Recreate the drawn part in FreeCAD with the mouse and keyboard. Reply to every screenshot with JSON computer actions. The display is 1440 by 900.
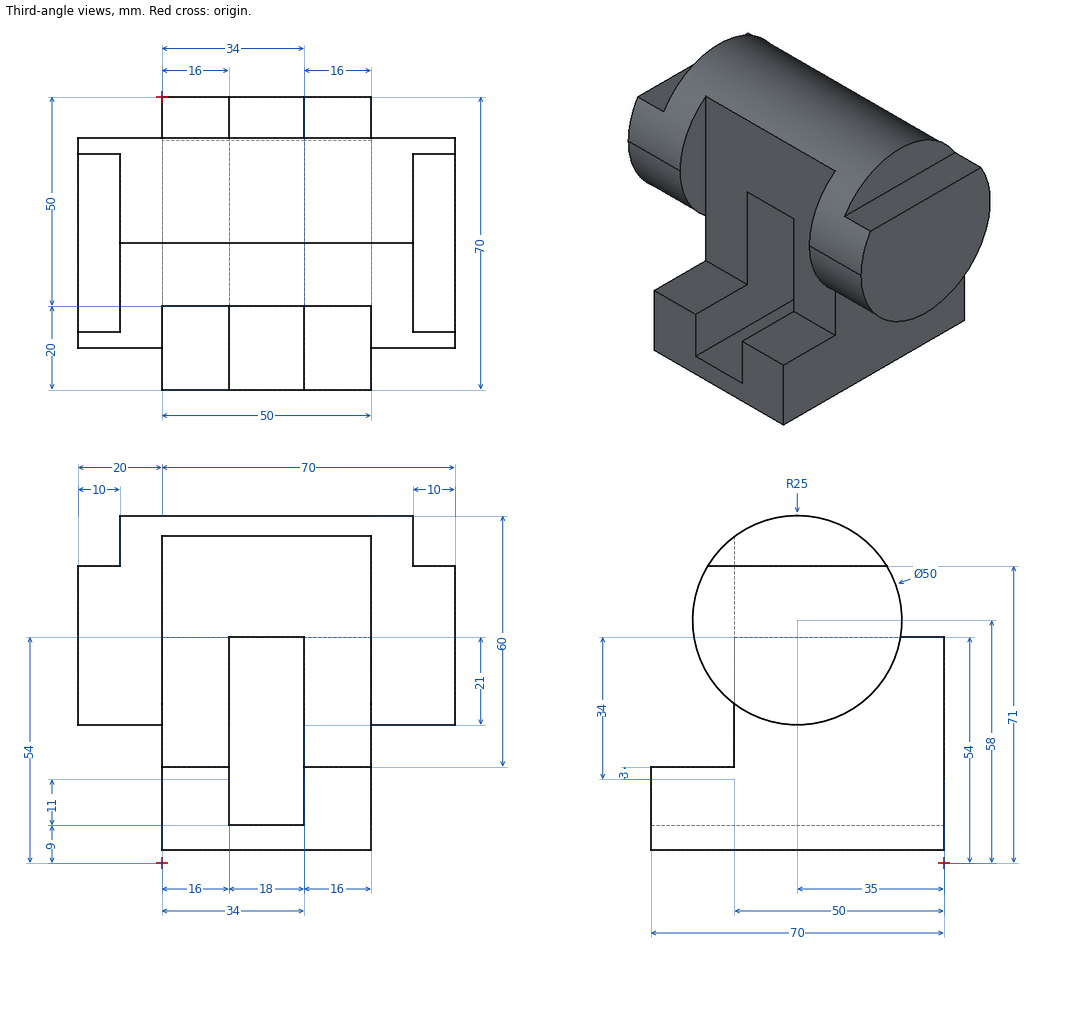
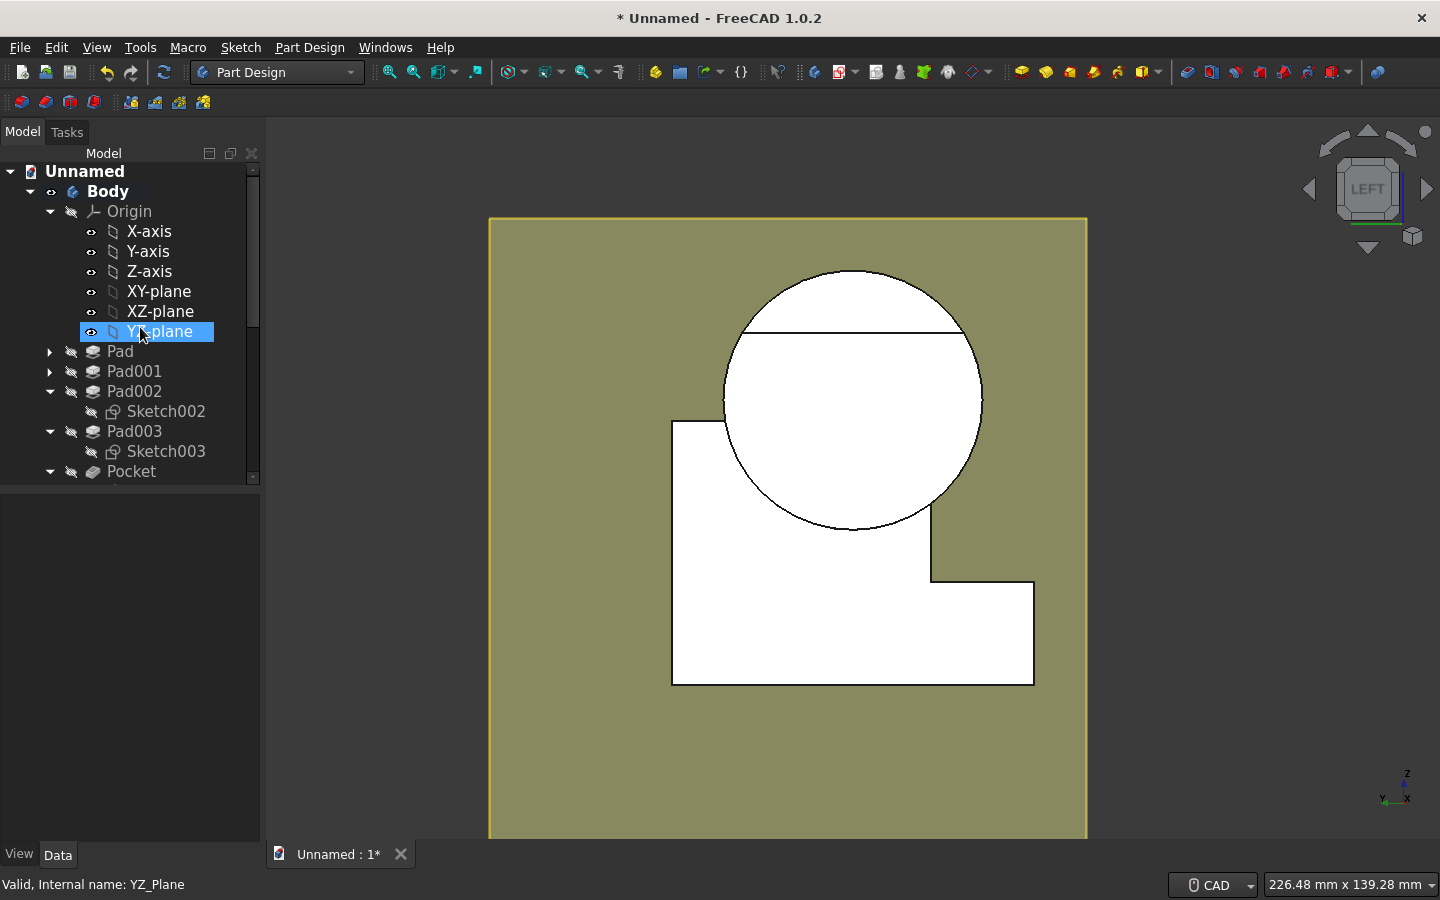
{"action": "scroll", "coordinate": [100, 327], "scroll_direction": "down", "scroll_amount": 6}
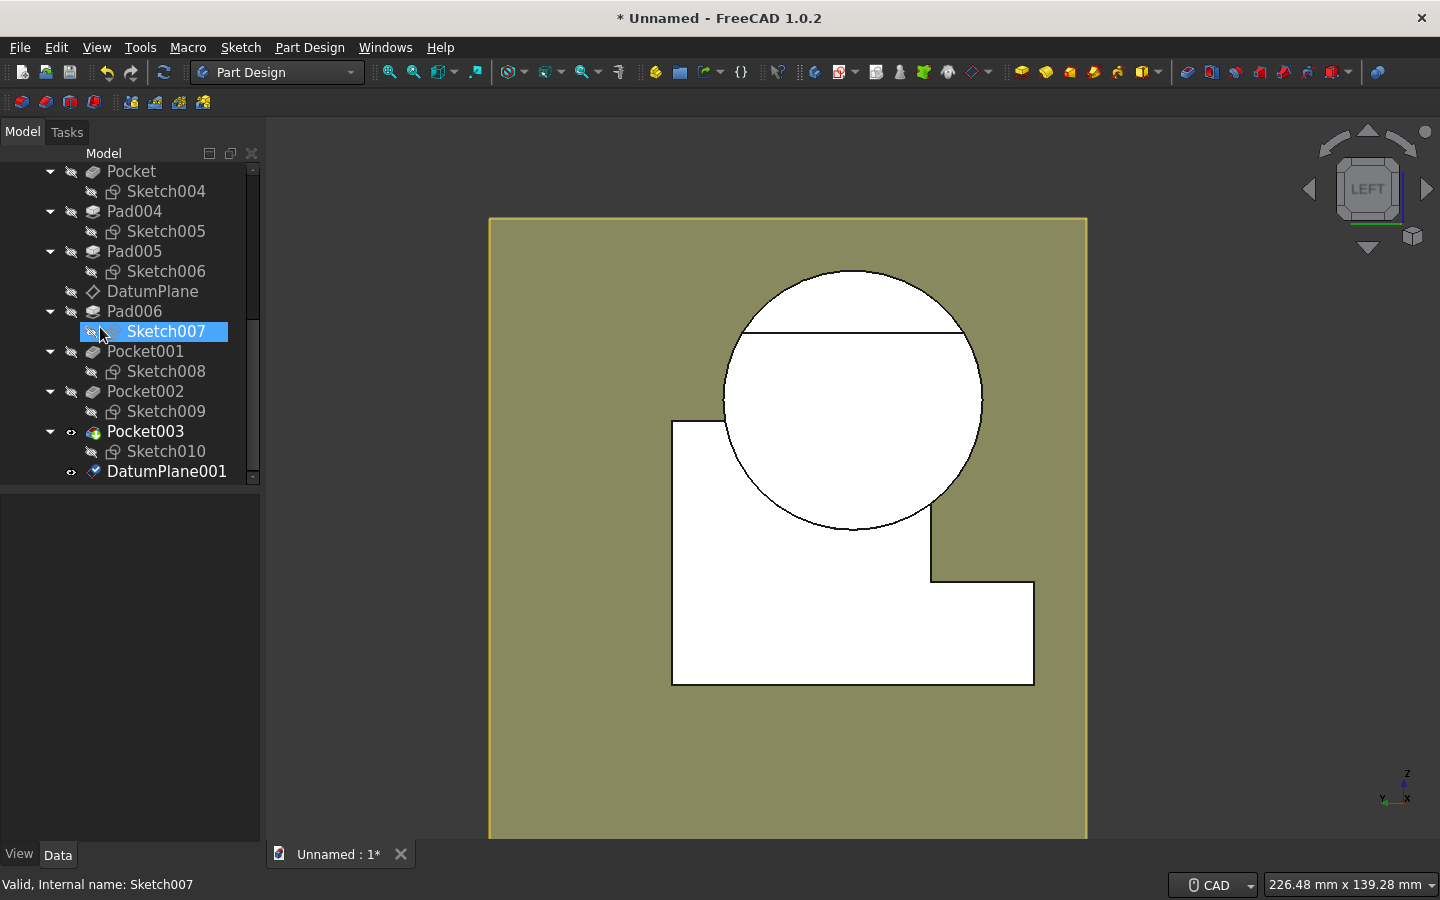
{"action": "left_click", "coordinate": [116, 472]}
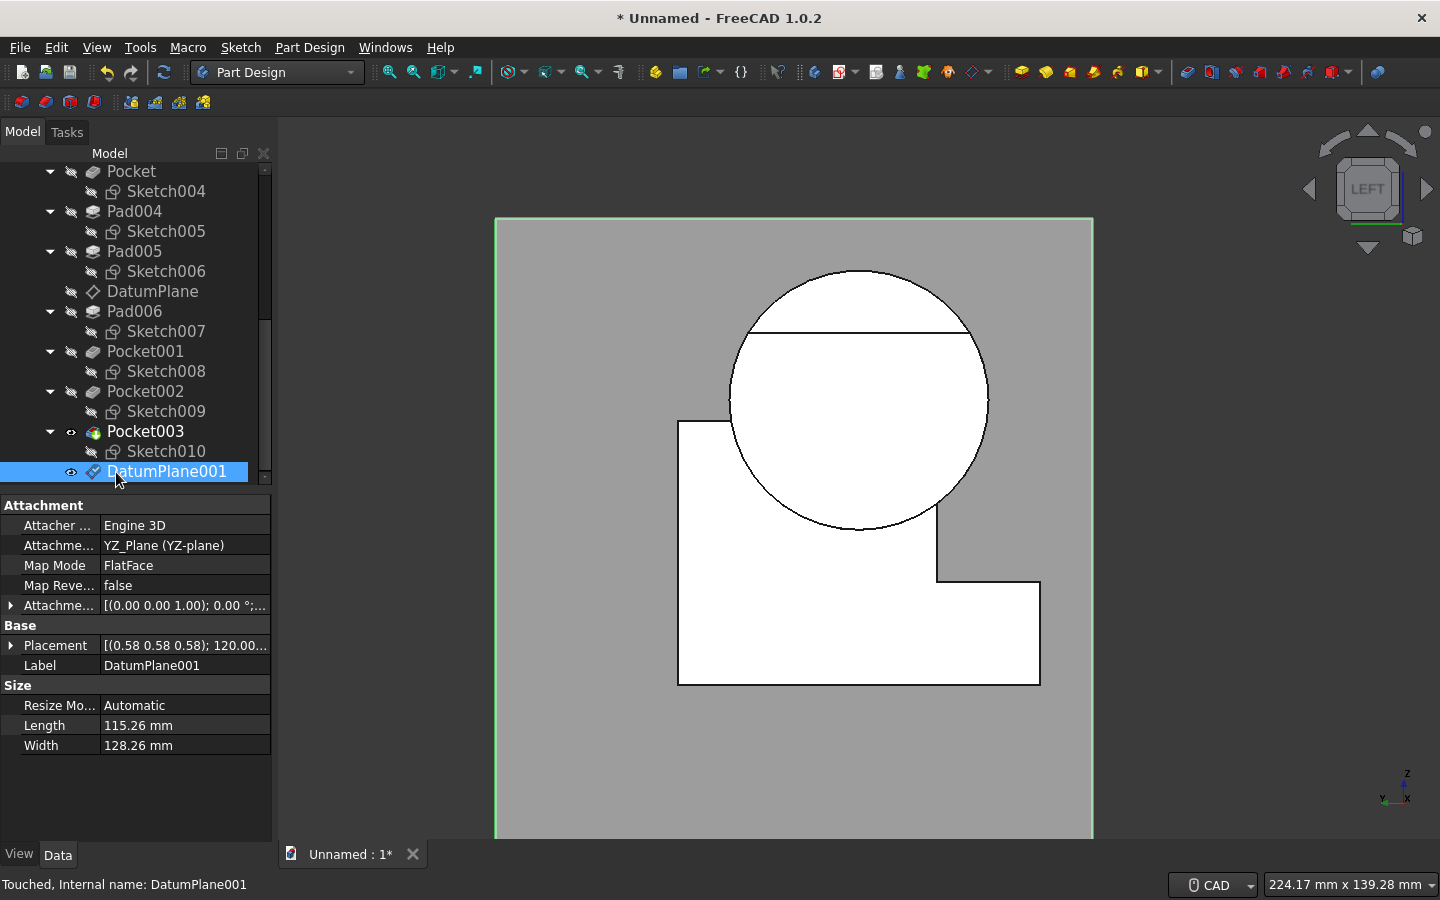
{"action": "left_click", "coordinate": [840, 72]}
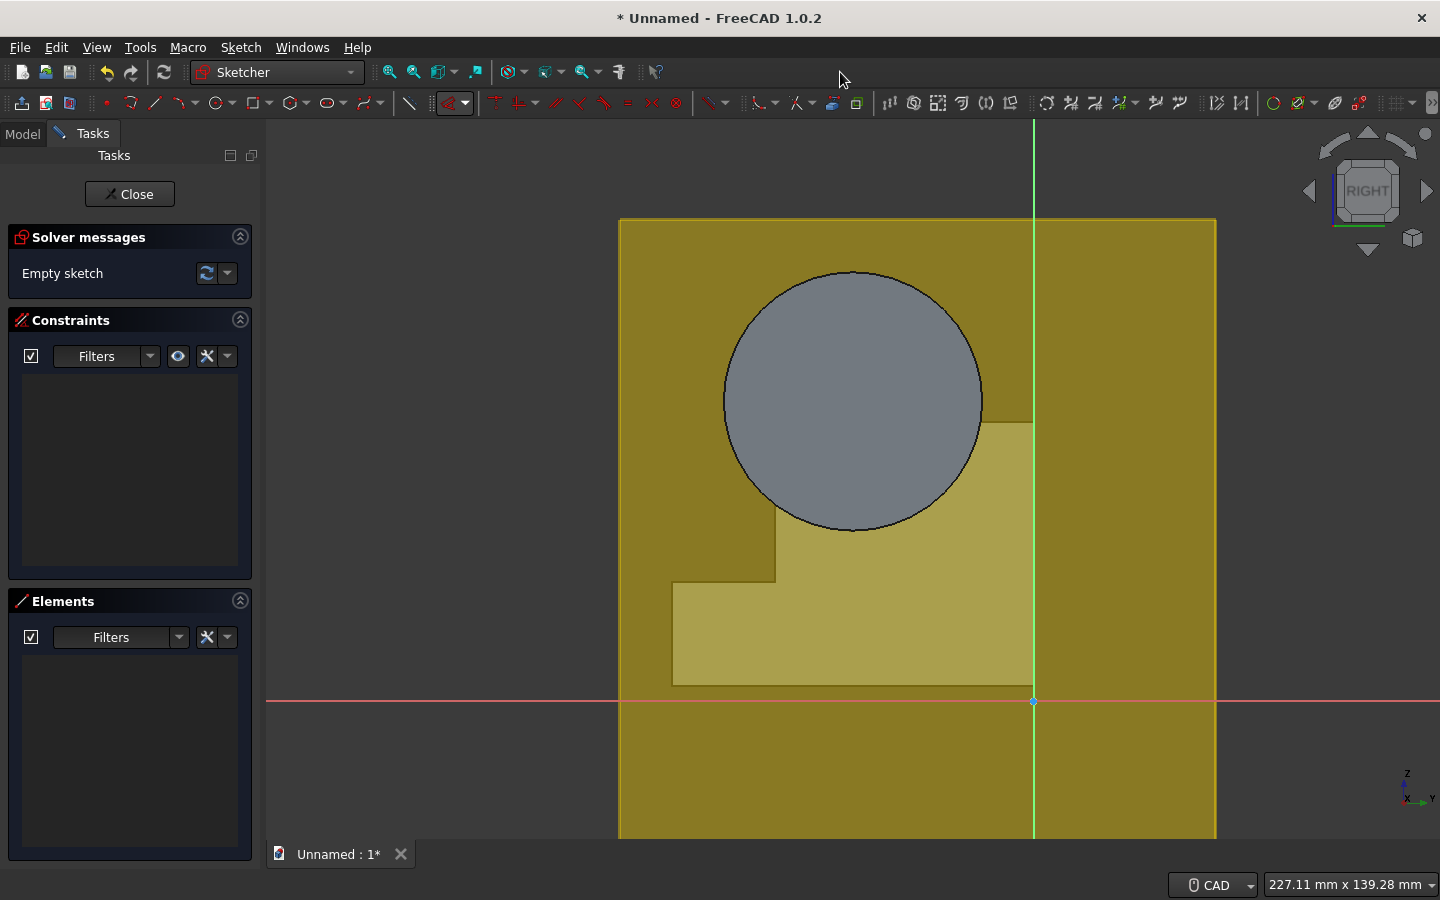
{"action": "key", "text": "q s"}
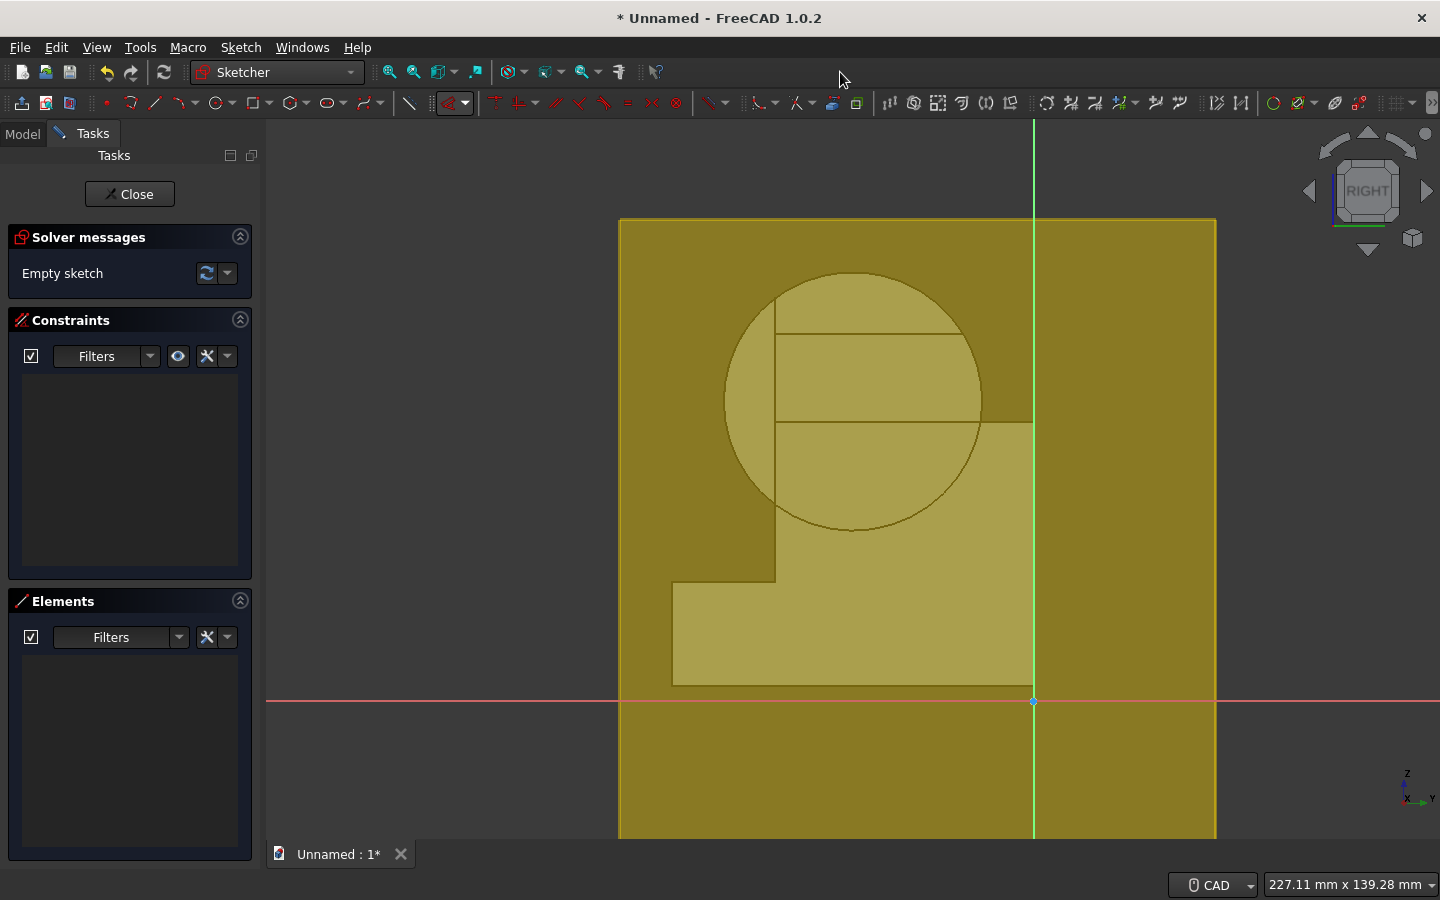
{"action": "key", "text": "g l"}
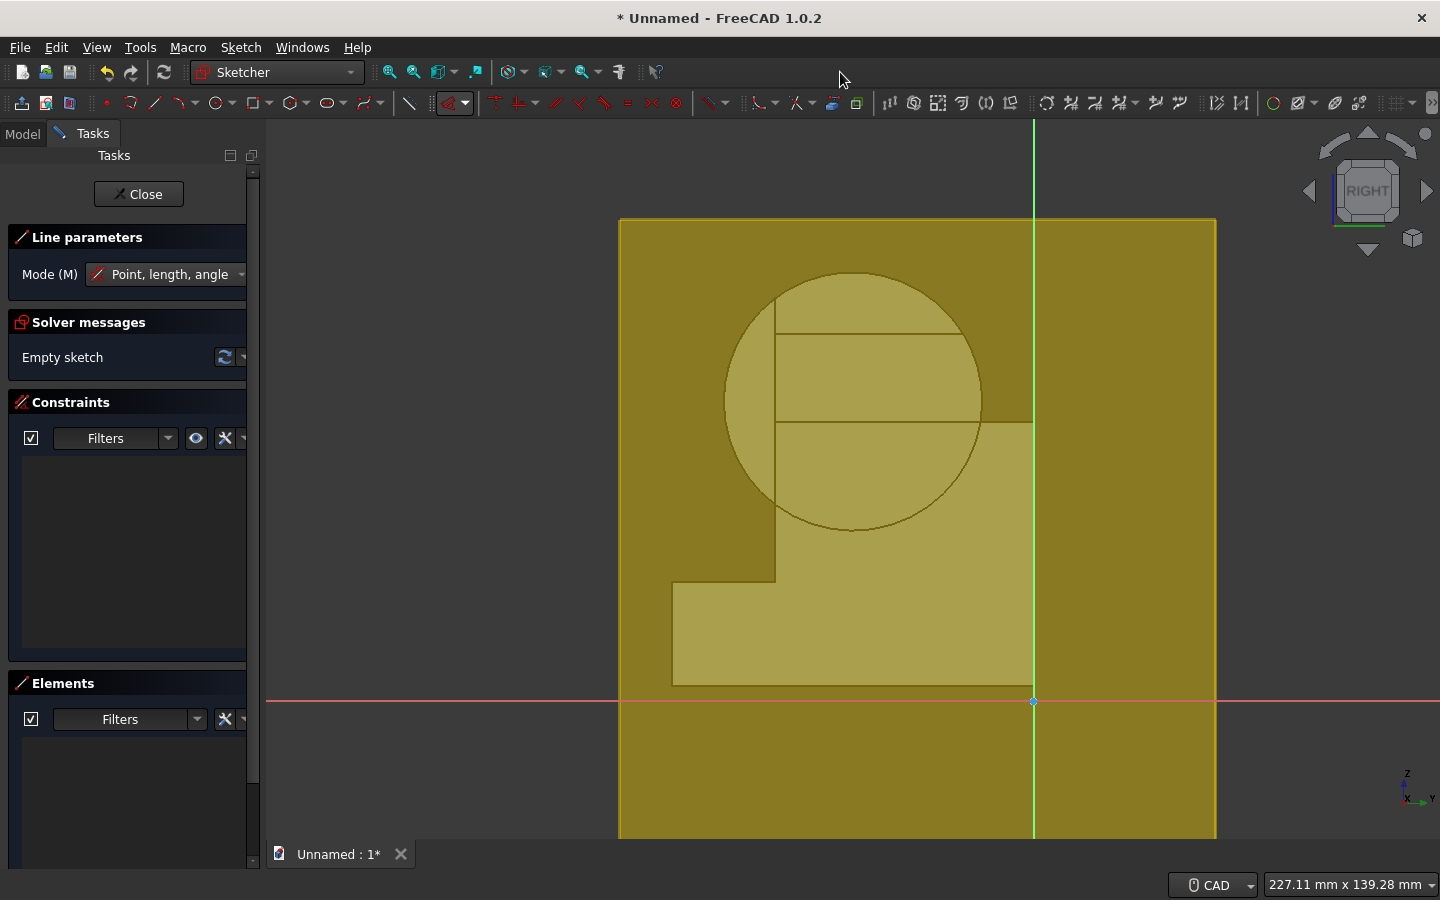
{"action": "left_click", "coordinate": [743, 334]}
{"action": "left_click", "coordinate": [963, 334]}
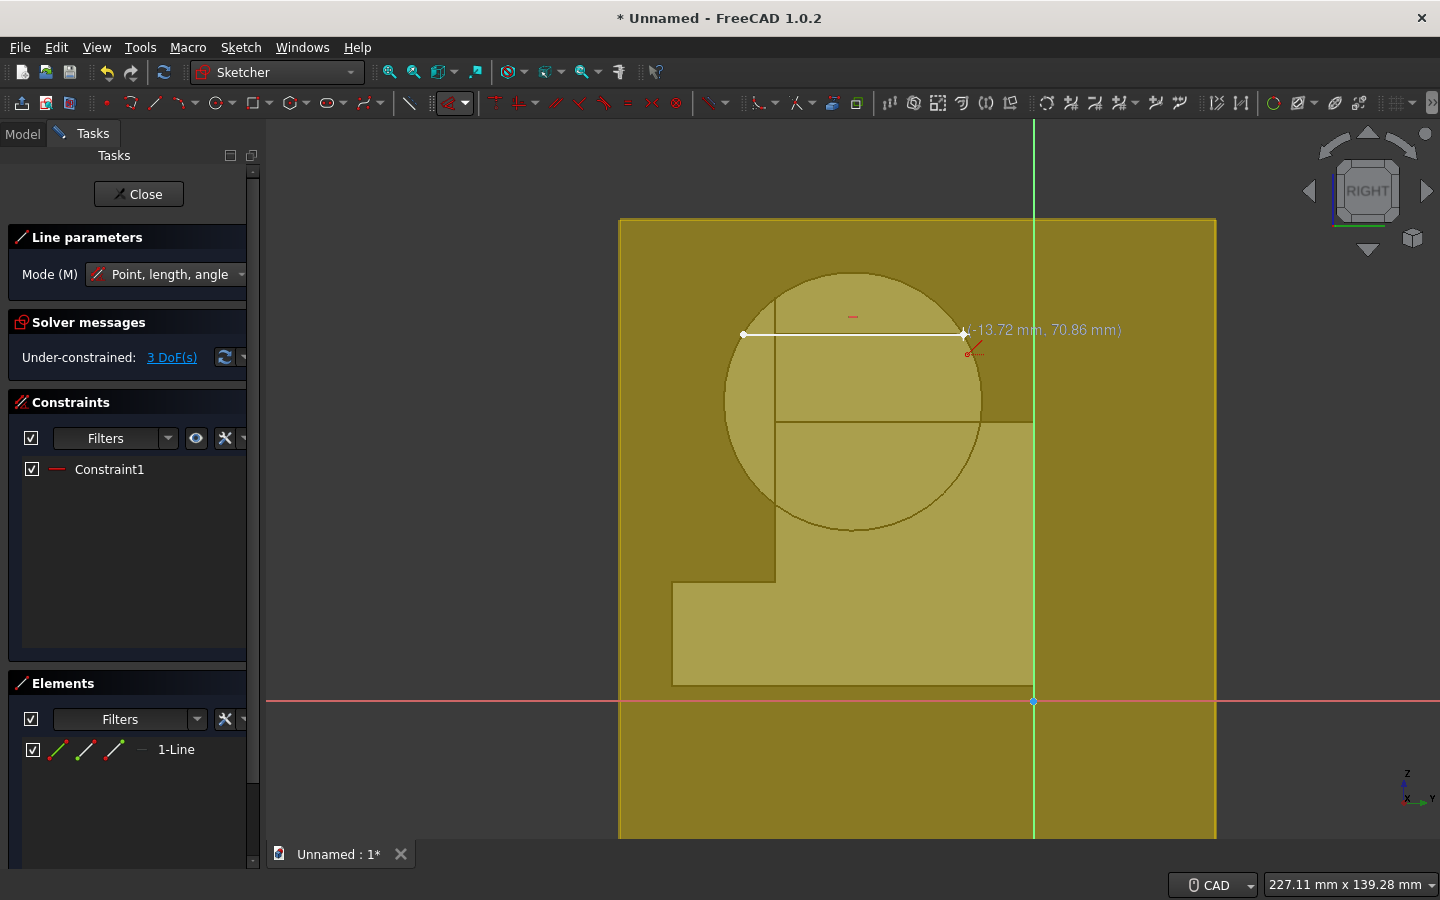
{"action": "key", "text": "g 3 a"}